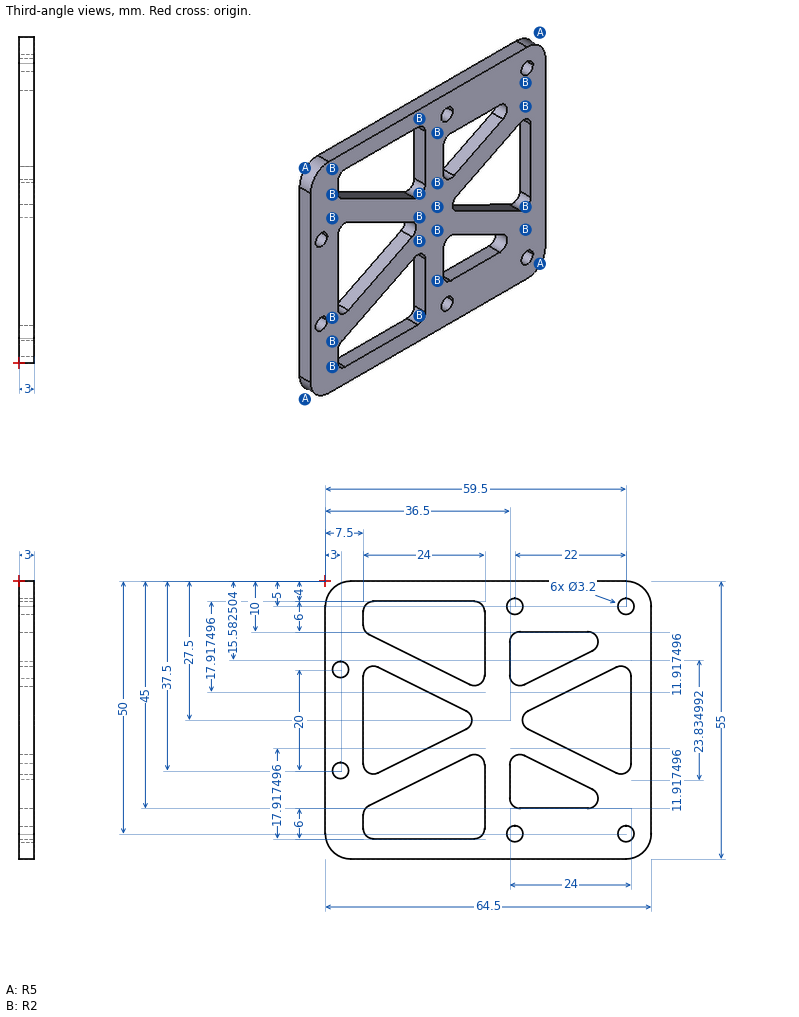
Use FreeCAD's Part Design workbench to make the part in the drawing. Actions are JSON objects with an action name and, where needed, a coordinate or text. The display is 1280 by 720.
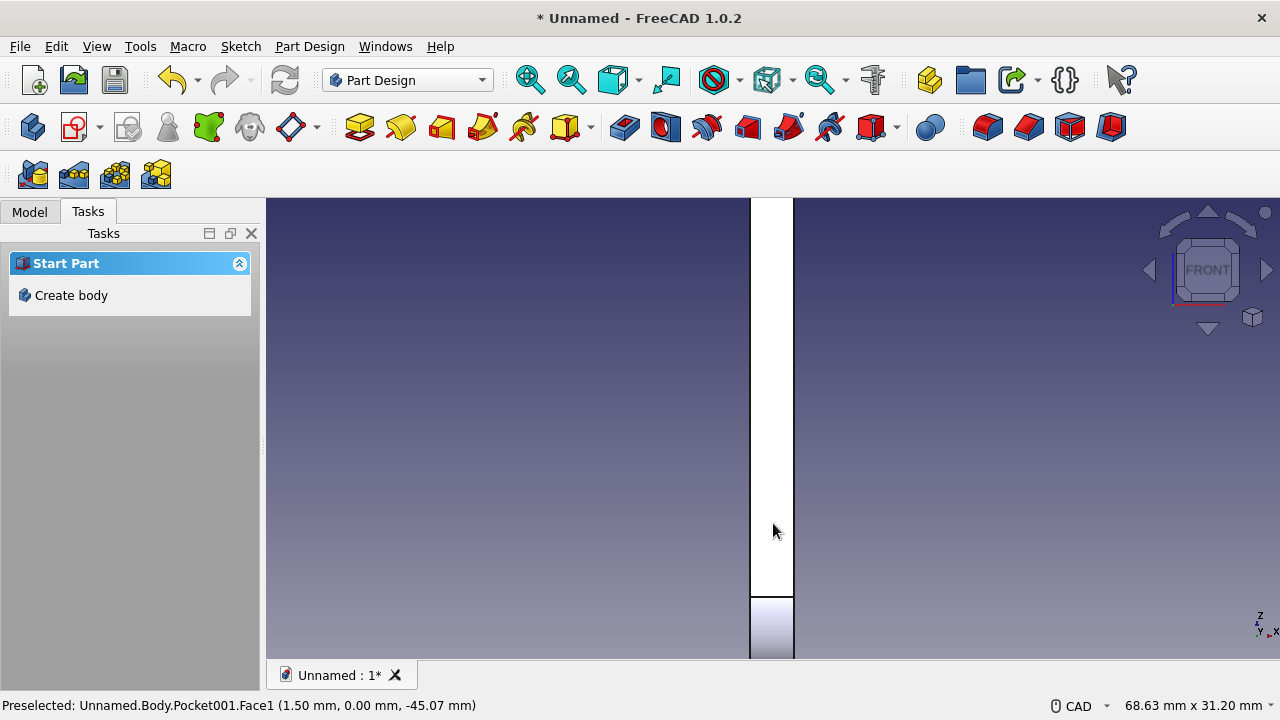
{"action": "key", "text": "v f"}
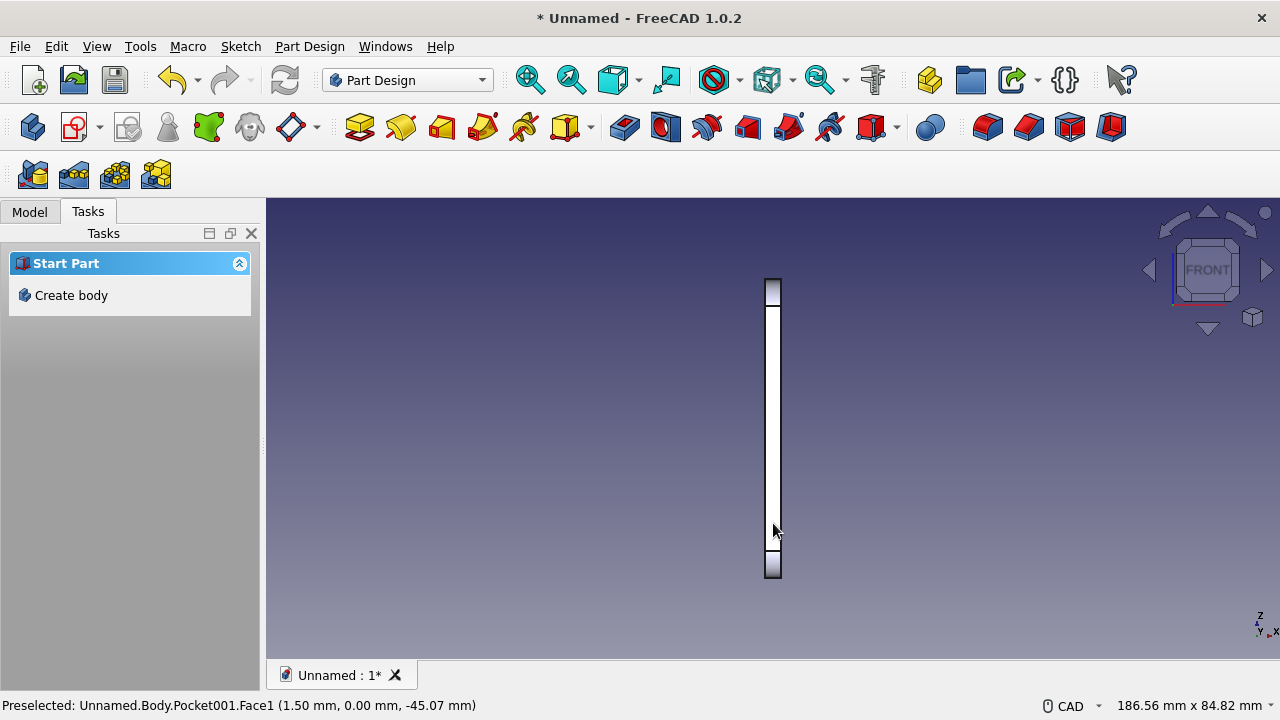
{"action": "key", "text": "3"}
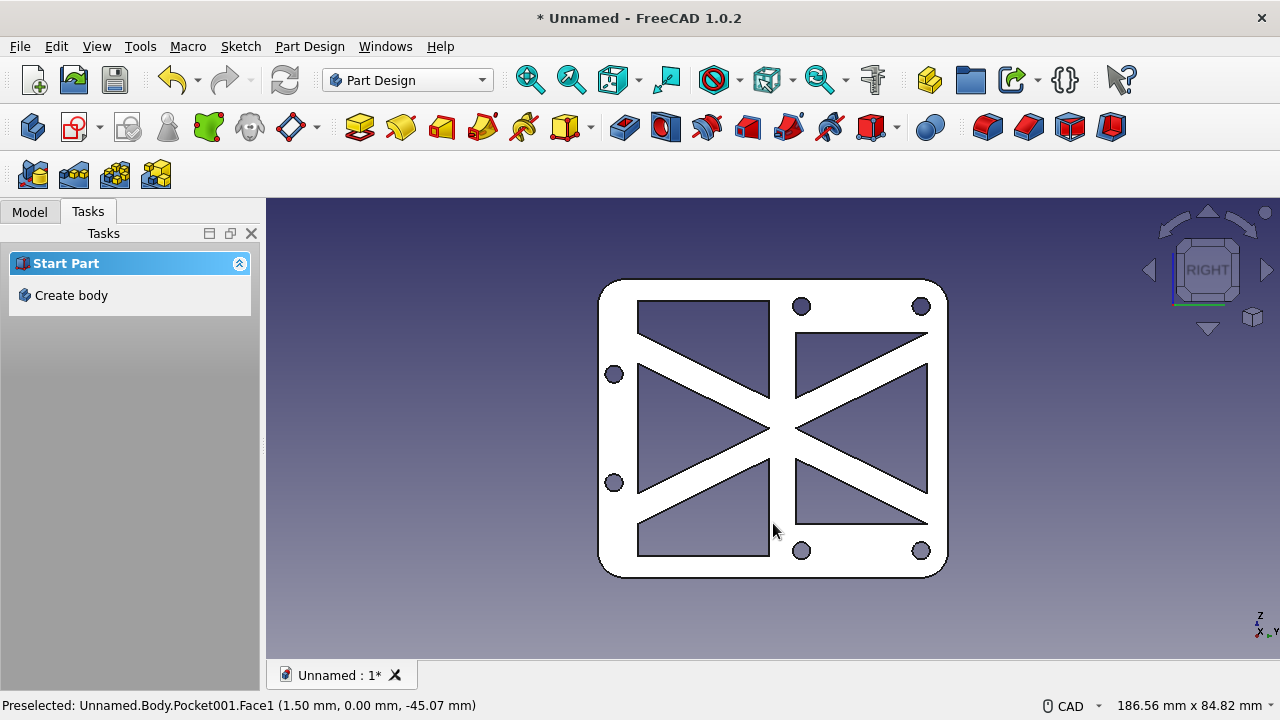
{"action": "scroll", "coordinate": [927, 523], "scroll_direction": "up", "scroll_amount": 5}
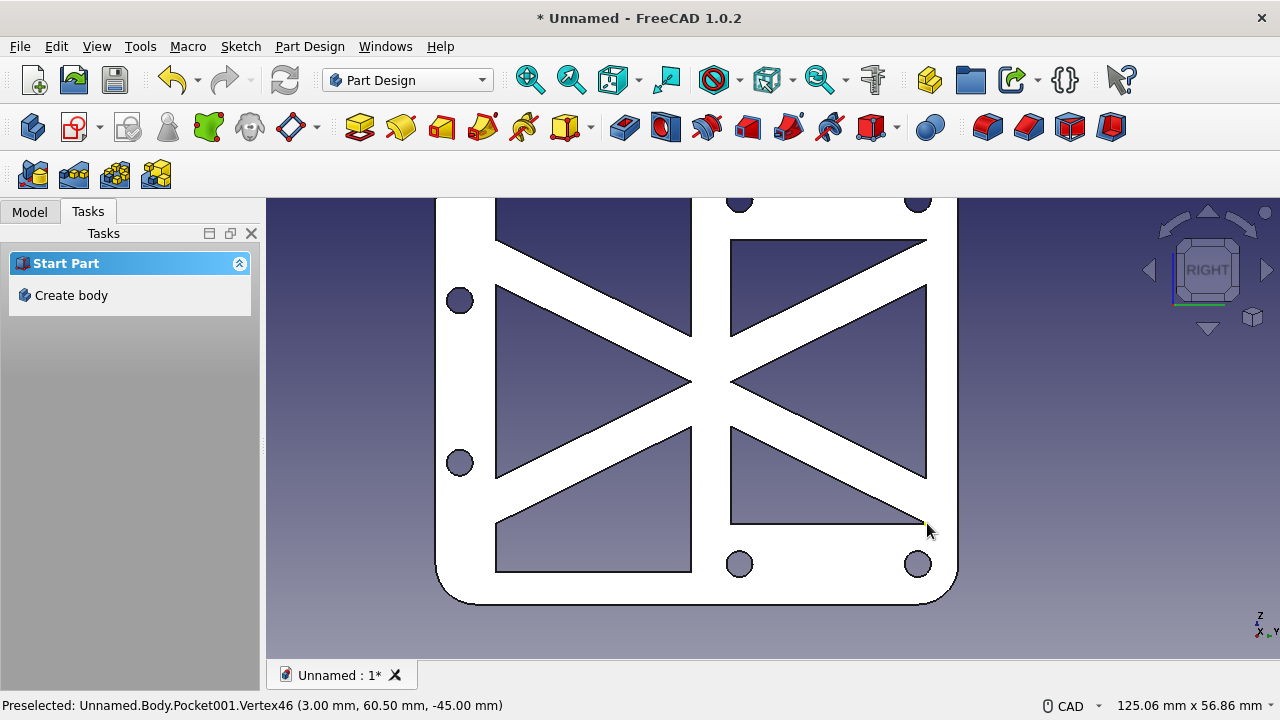
{"action": "left_click", "coordinate": [531, 80]}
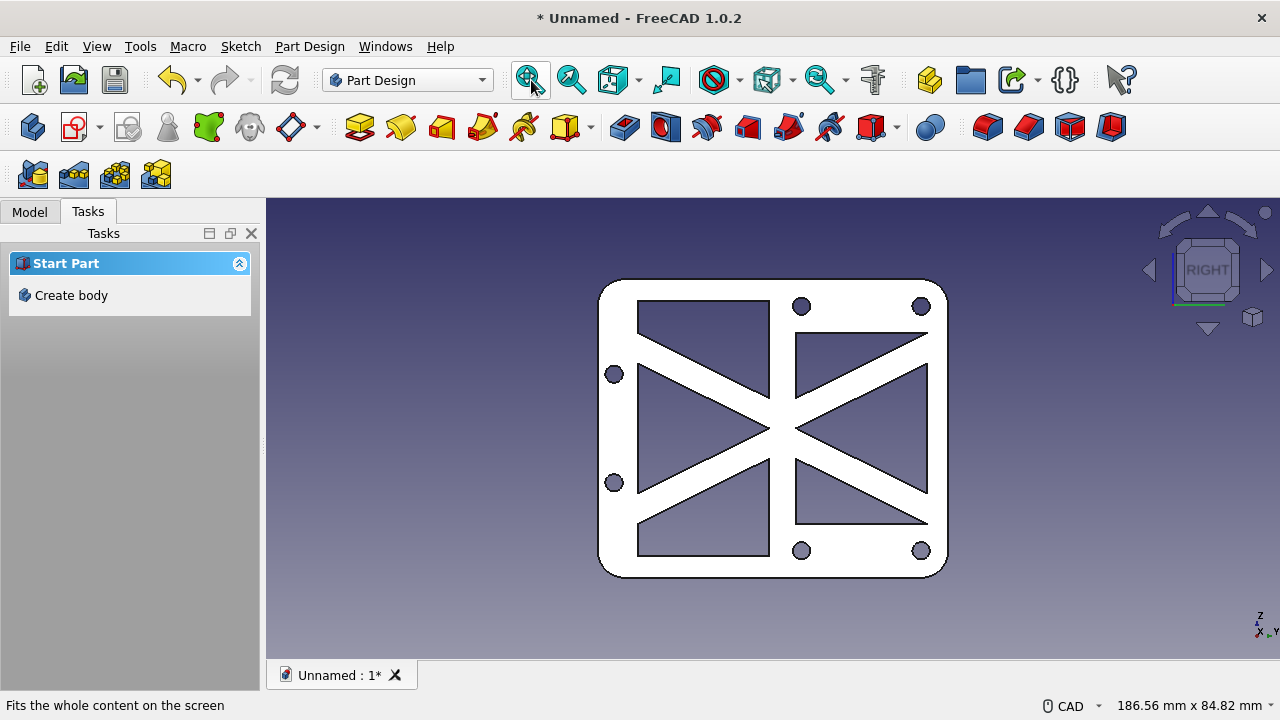
{"action": "key", "text": "5"}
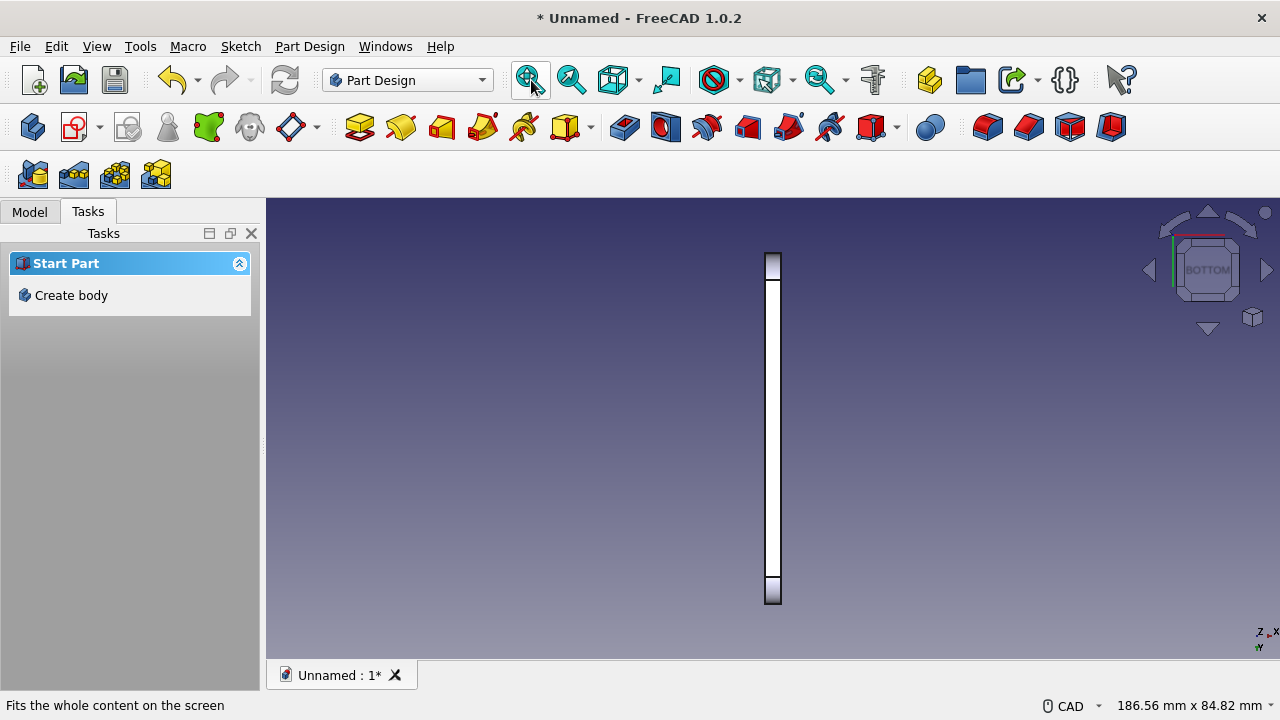
{"action": "scroll", "coordinate": [773, 581], "scroll_direction": "up", "scroll_amount": 5}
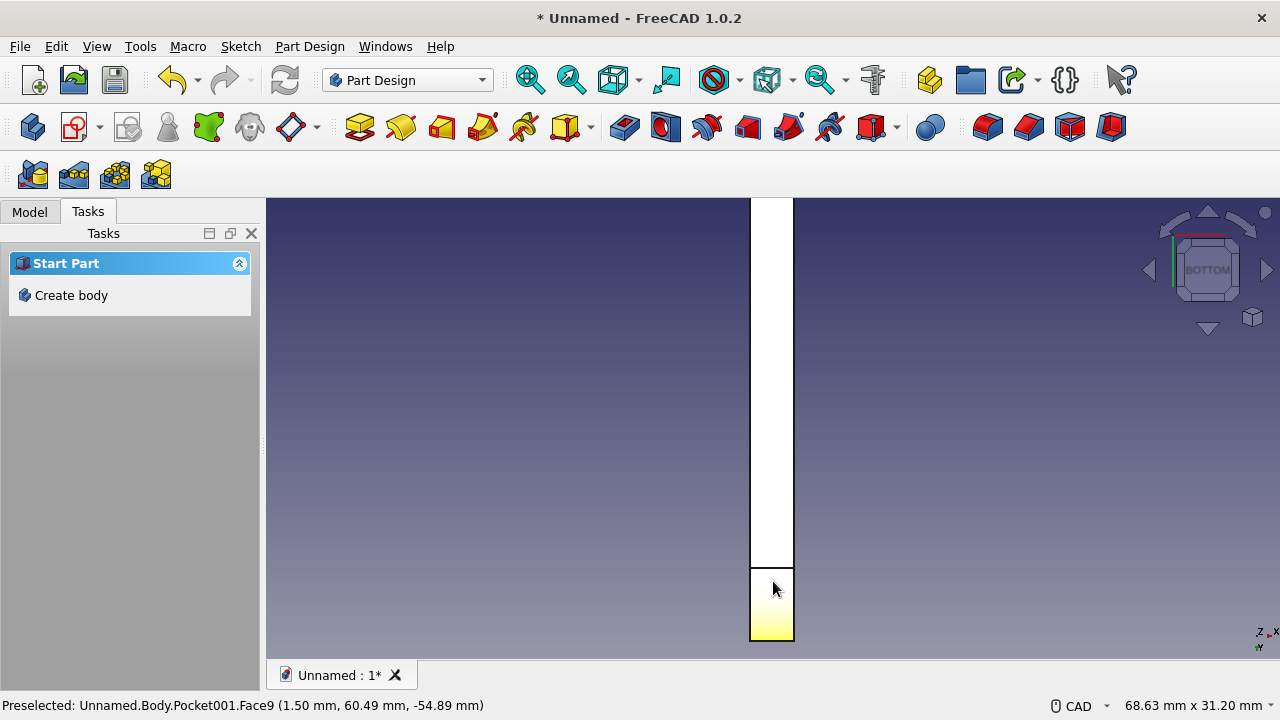
{"action": "left_click", "coordinate": [531, 80]}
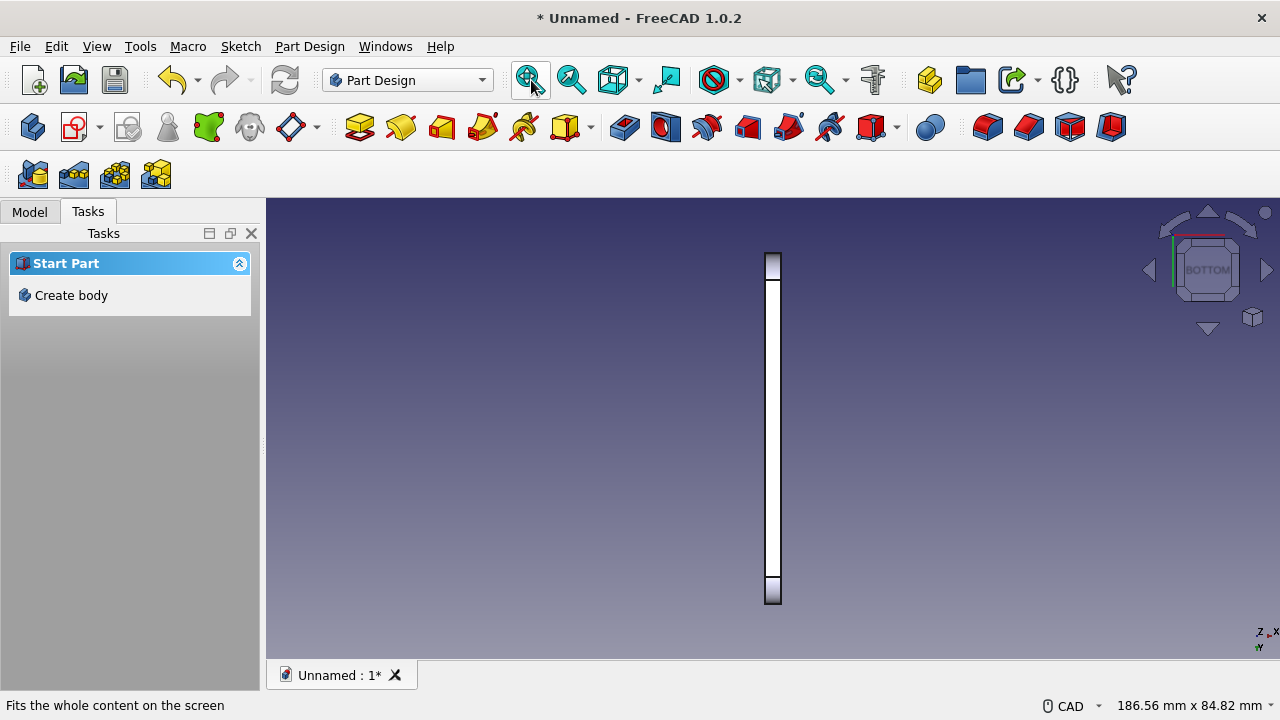
{"action": "key", "text": "4"}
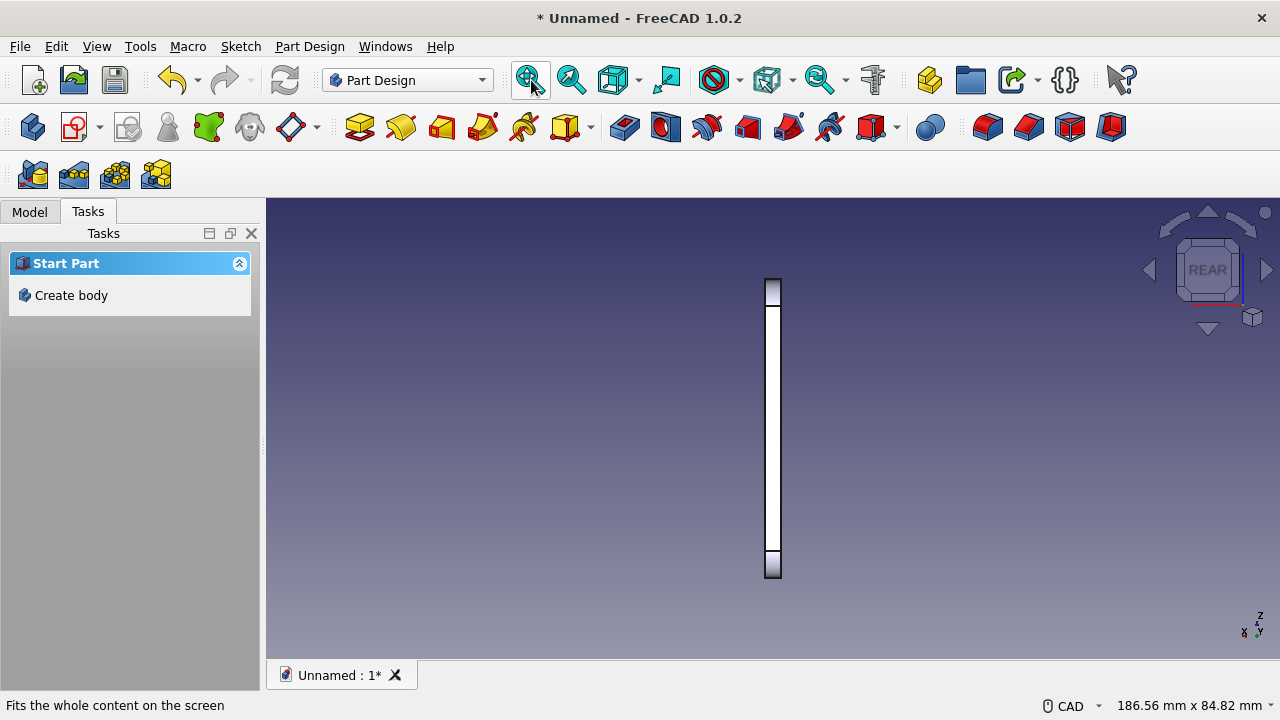
{"action": "scroll", "coordinate": [773, 523], "scroll_direction": "up", "scroll_amount": 5}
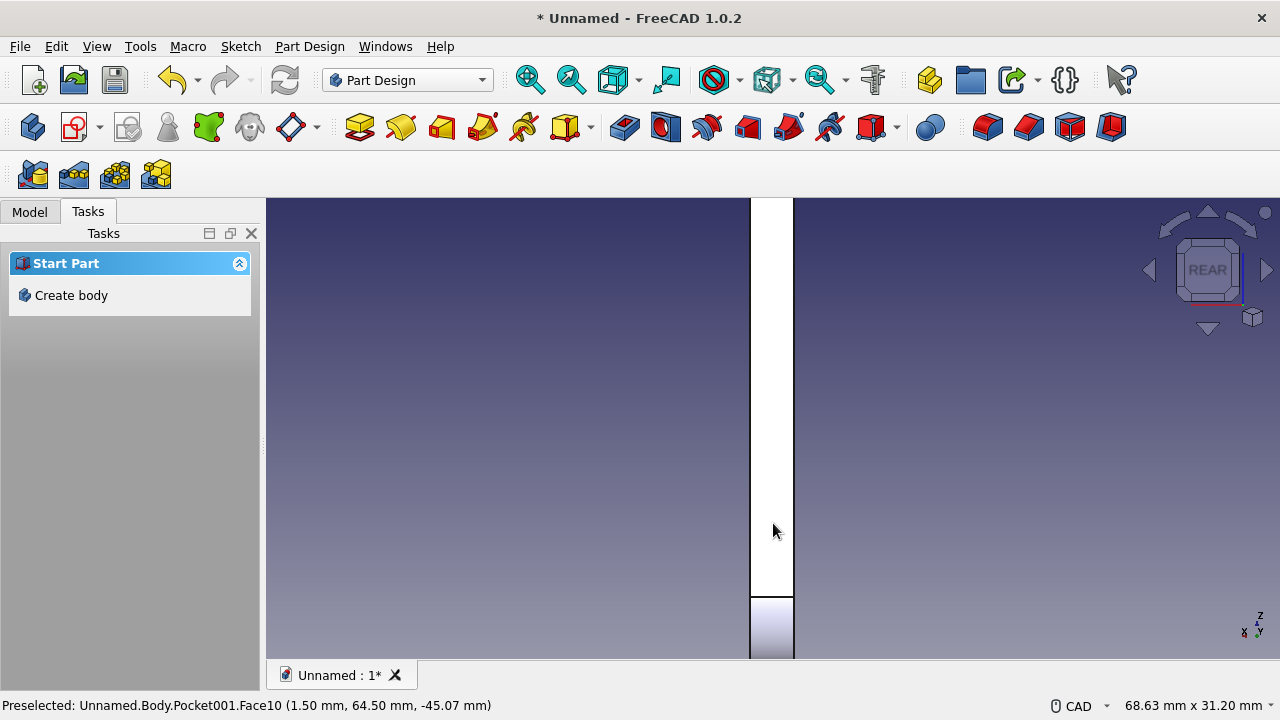
{"action": "left_click", "coordinate": [531, 80]}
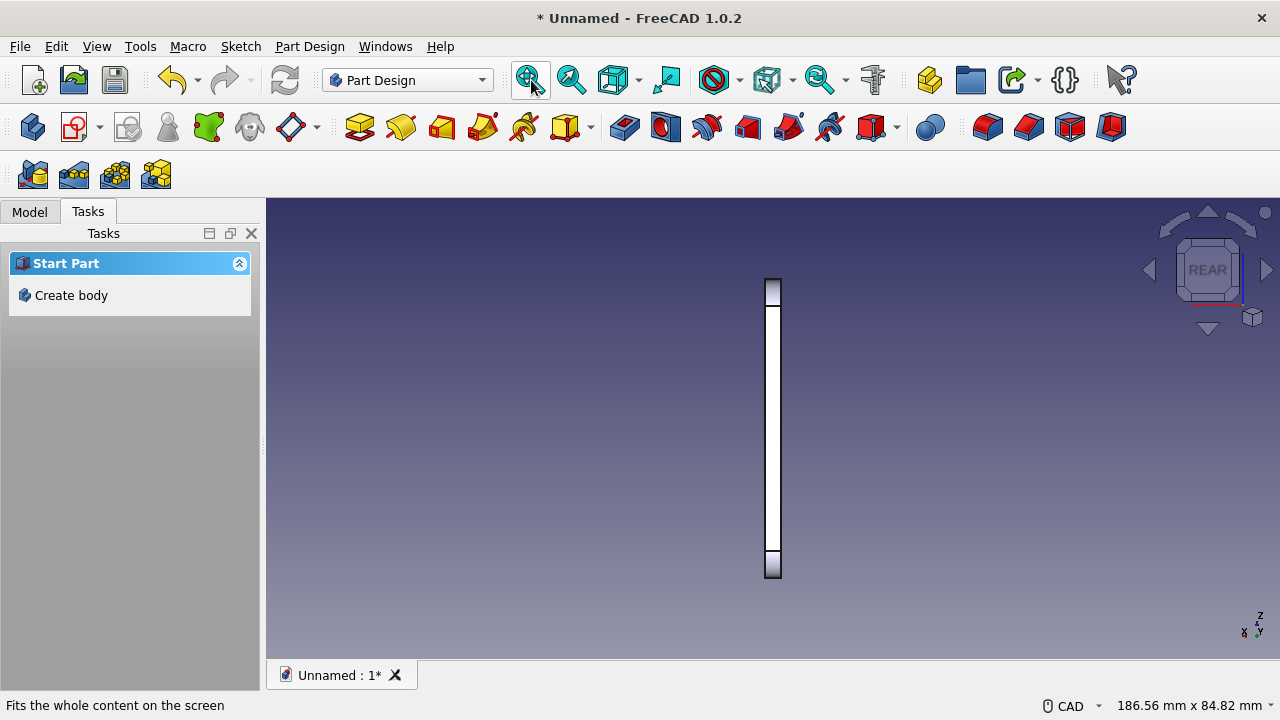
{"action": "key", "text": "6"}